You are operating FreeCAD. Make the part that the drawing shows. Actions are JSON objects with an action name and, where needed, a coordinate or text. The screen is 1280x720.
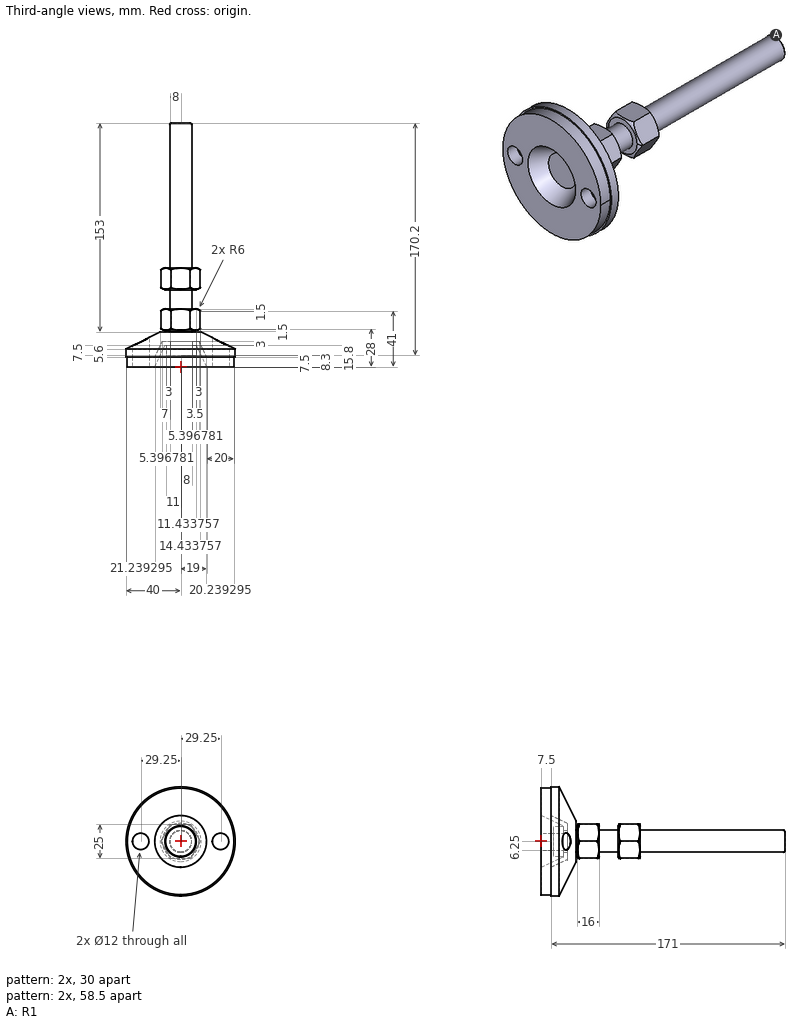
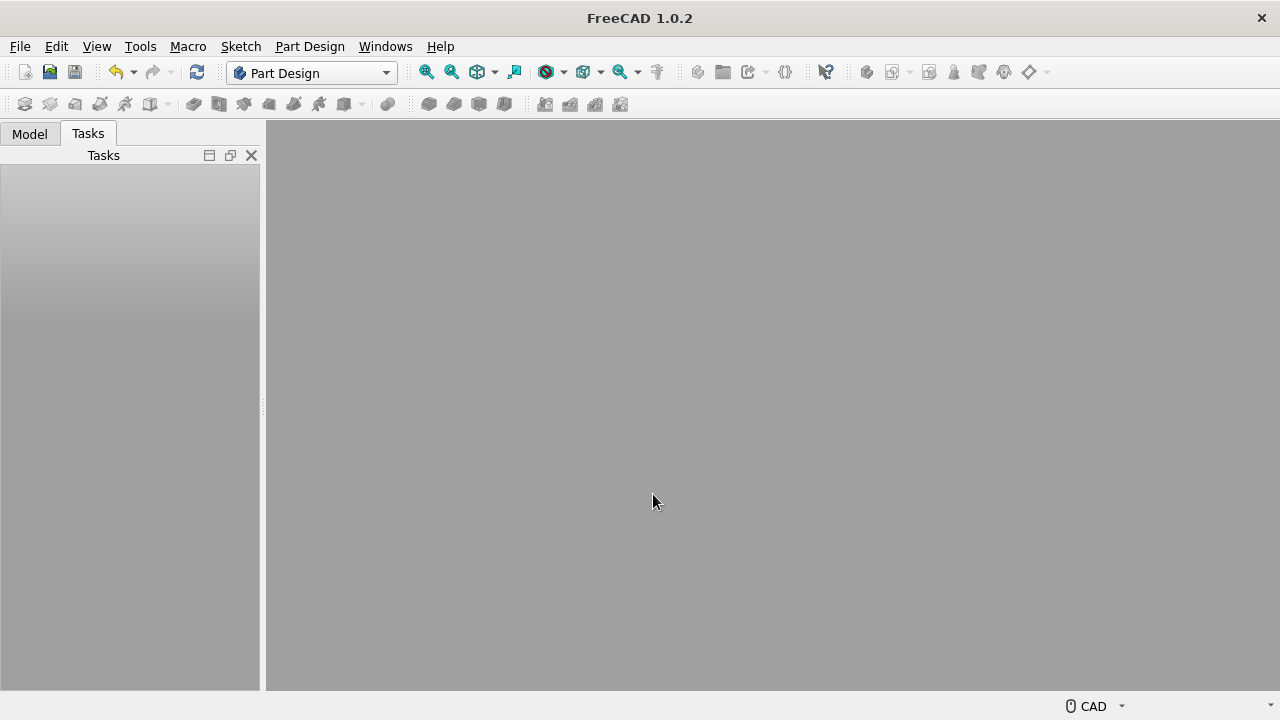
{"action": "left_click", "coordinate": [25, 72]}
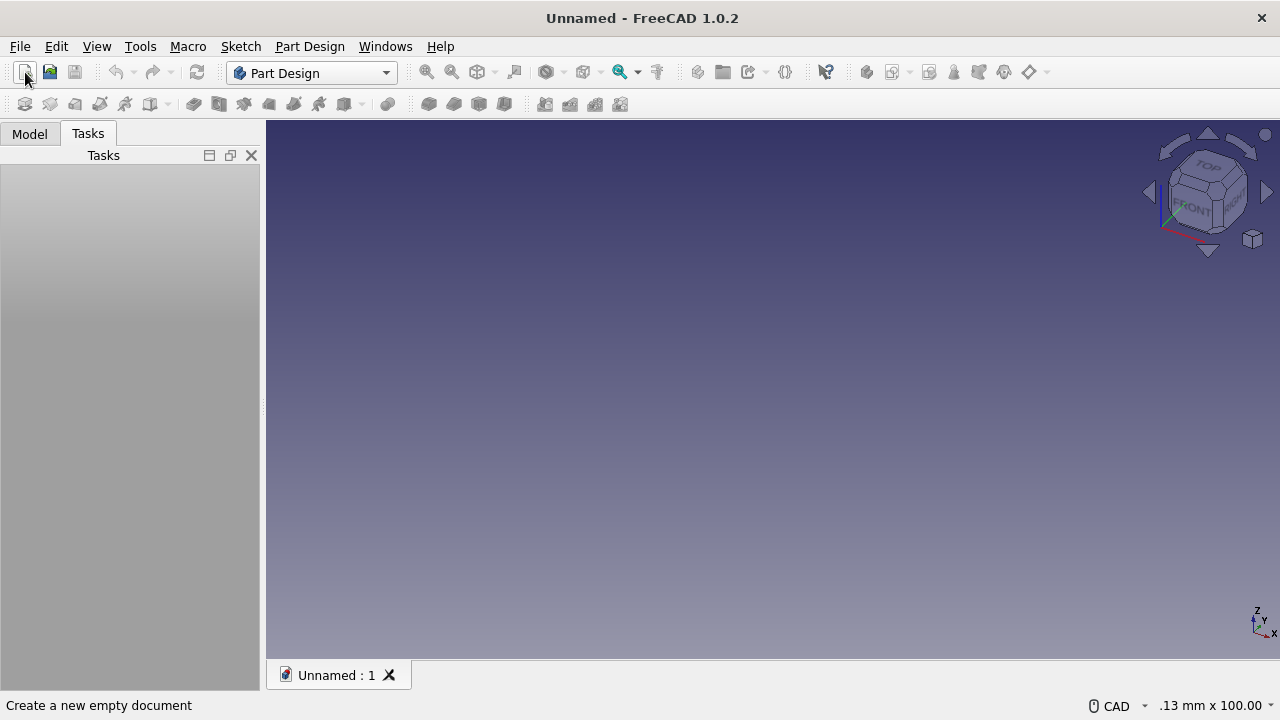
{"action": "left_click", "coordinate": [892, 72]}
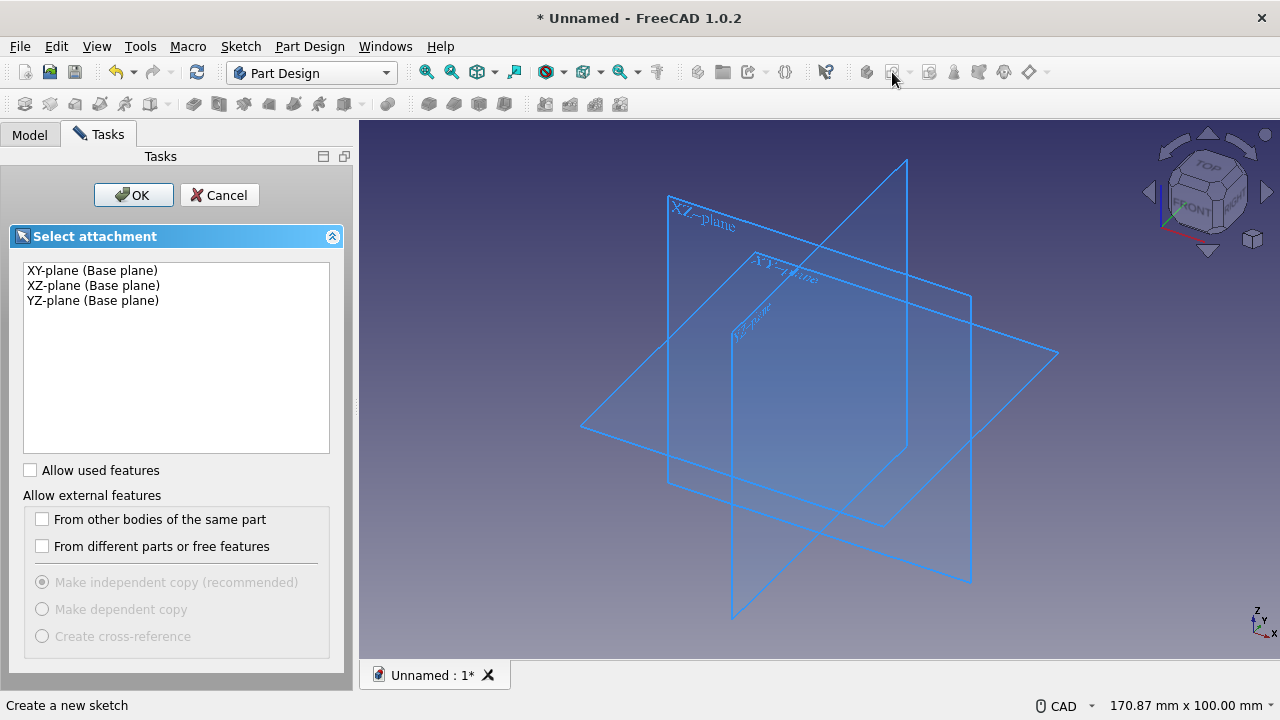
{"action": "left_click", "coordinate": [84, 270]}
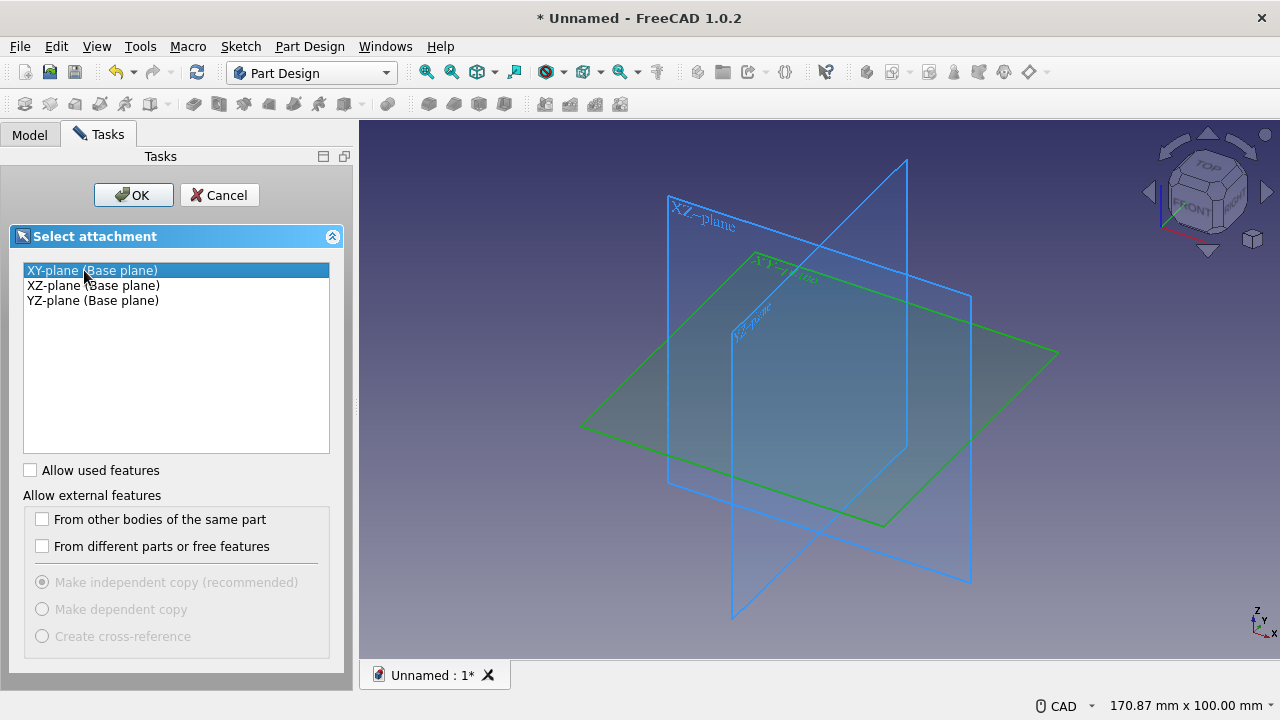
{"action": "left_click", "coordinate": [134, 195]}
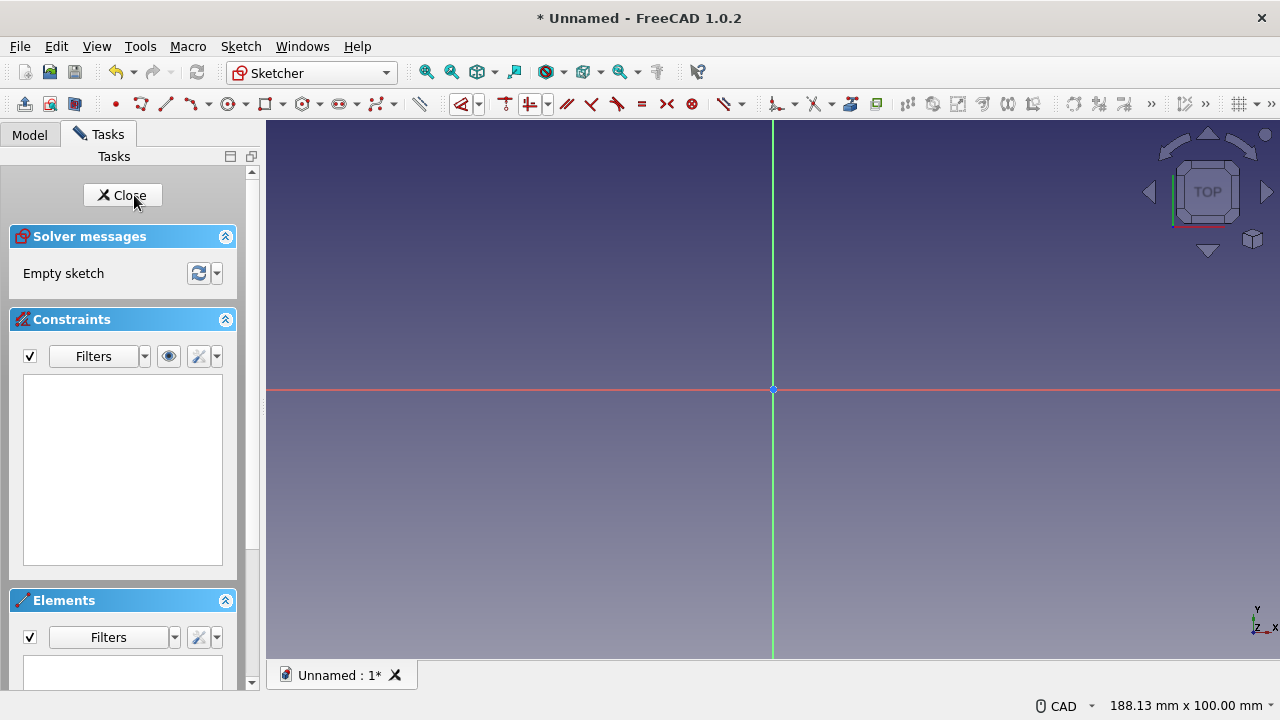
{"action": "scroll", "coordinate": [979, 309], "scroll_direction": "up", "scroll_amount": 5}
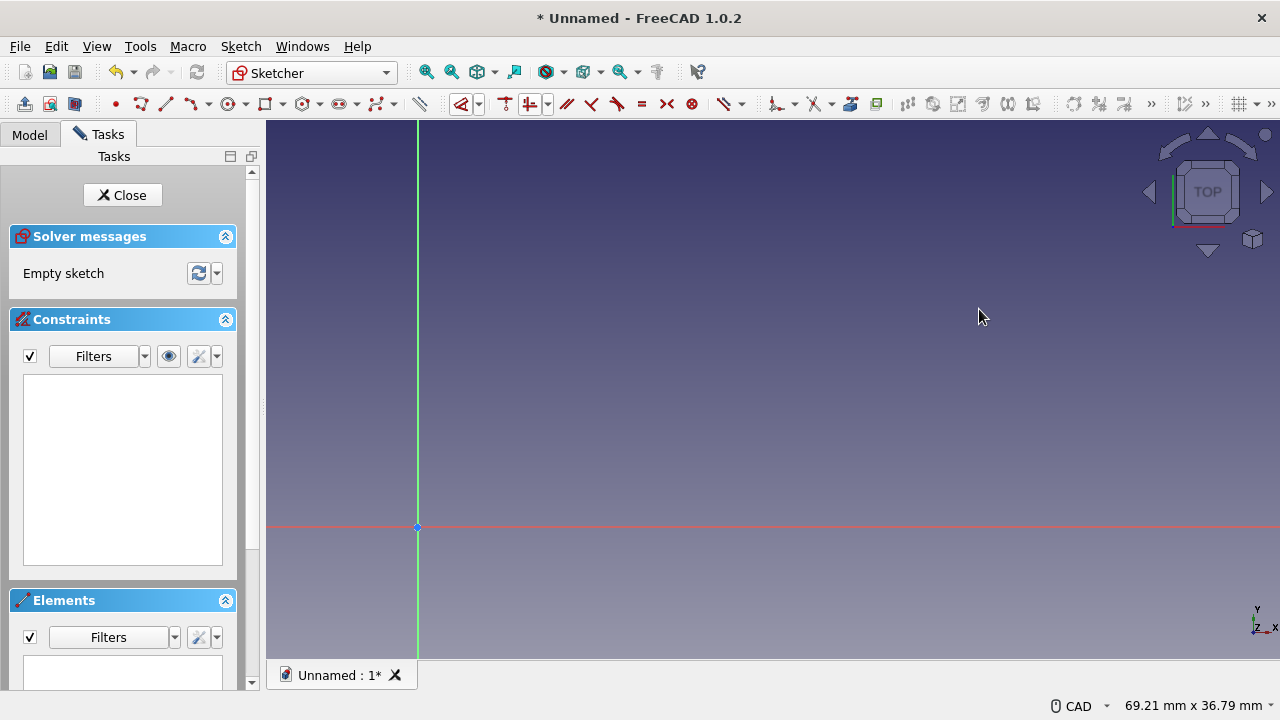
{"action": "left_click", "coordinate": [141, 104]}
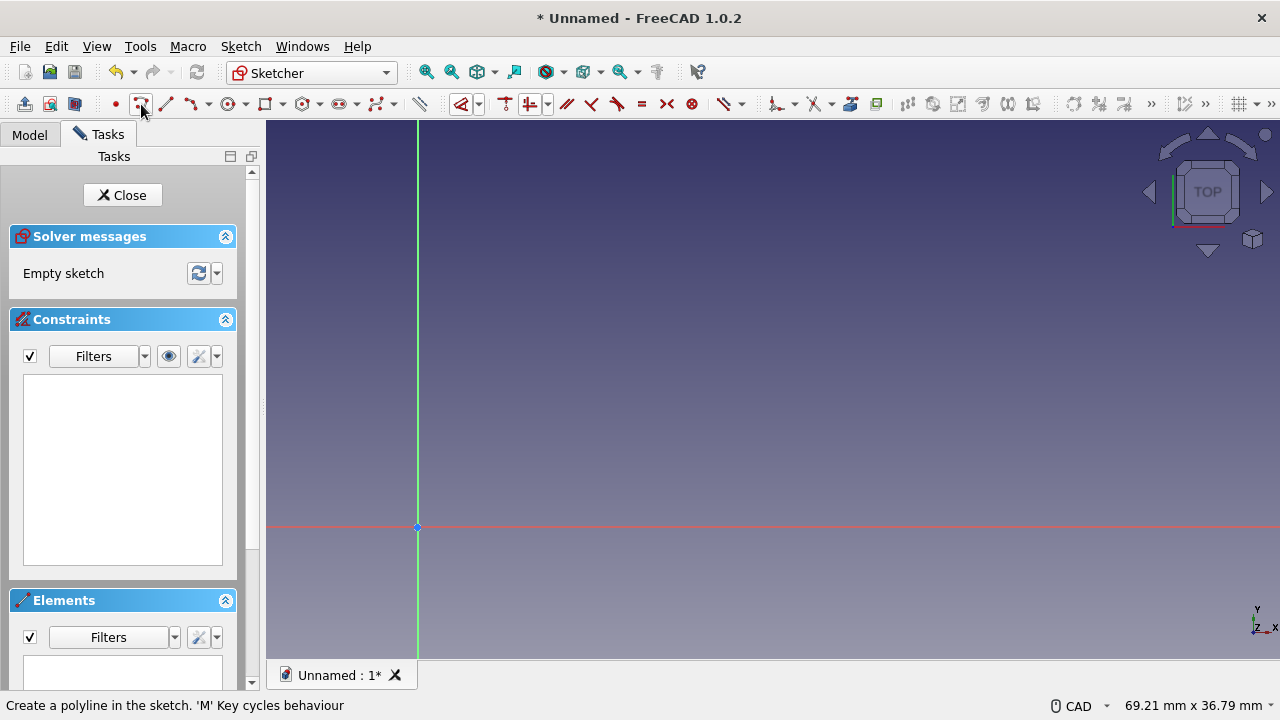
{"action": "left_click", "coordinate": [535, 296]}
{"action": "left_click", "coordinate": [586, 296]}
{"action": "left_click", "coordinate": [696, 527]}
{"action": "left_click", "coordinate": [989, 518]}
{"action": "left_click", "coordinate": [989, 417]}
{"action": "left_click", "coordinate": [693, 417]}
{"action": "left_click", "coordinate": [614, 252]}
{"action": "left_click", "coordinate": [535, 252]}
{"action": "left_click", "coordinate": [535, 297]}
{"action": "key", "text": "Escape"}
{"action": "key", "text": "Escape"}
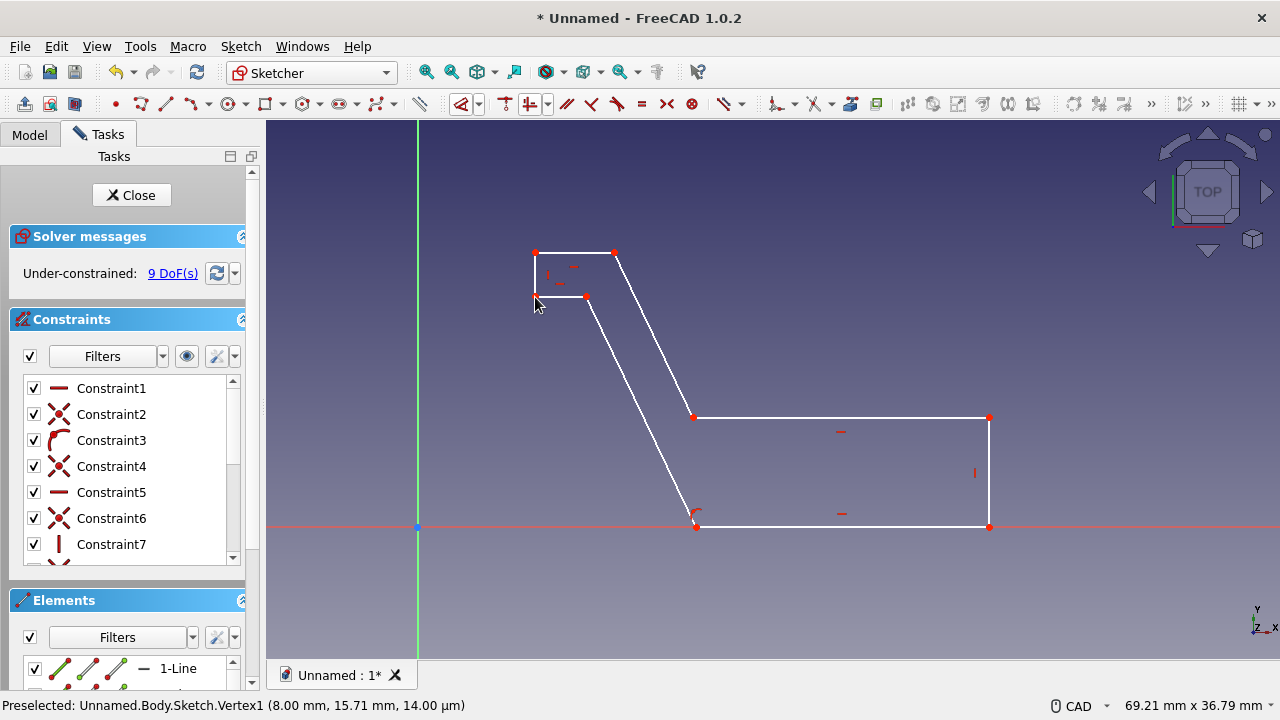
{"action": "left_click", "coordinate": [460, 104]}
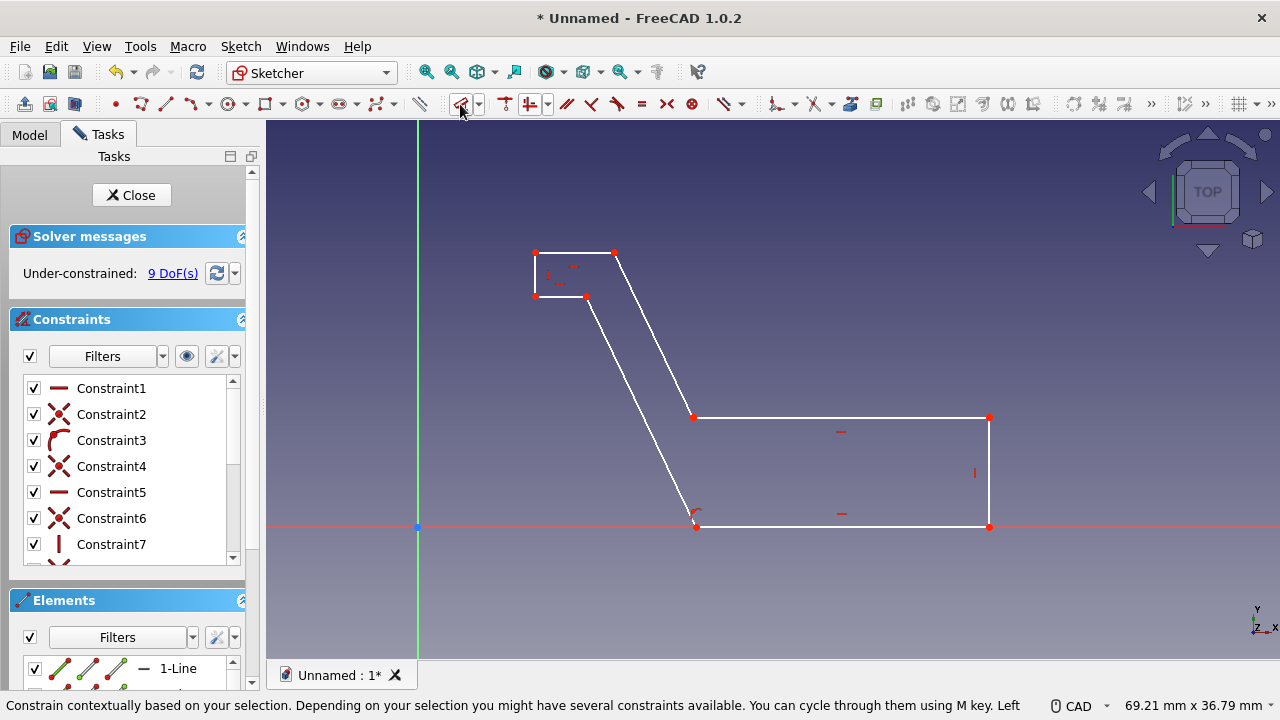
{"action": "left_click", "coordinate": [535, 266]}
{"action": "left_click", "coordinate": [501, 275]}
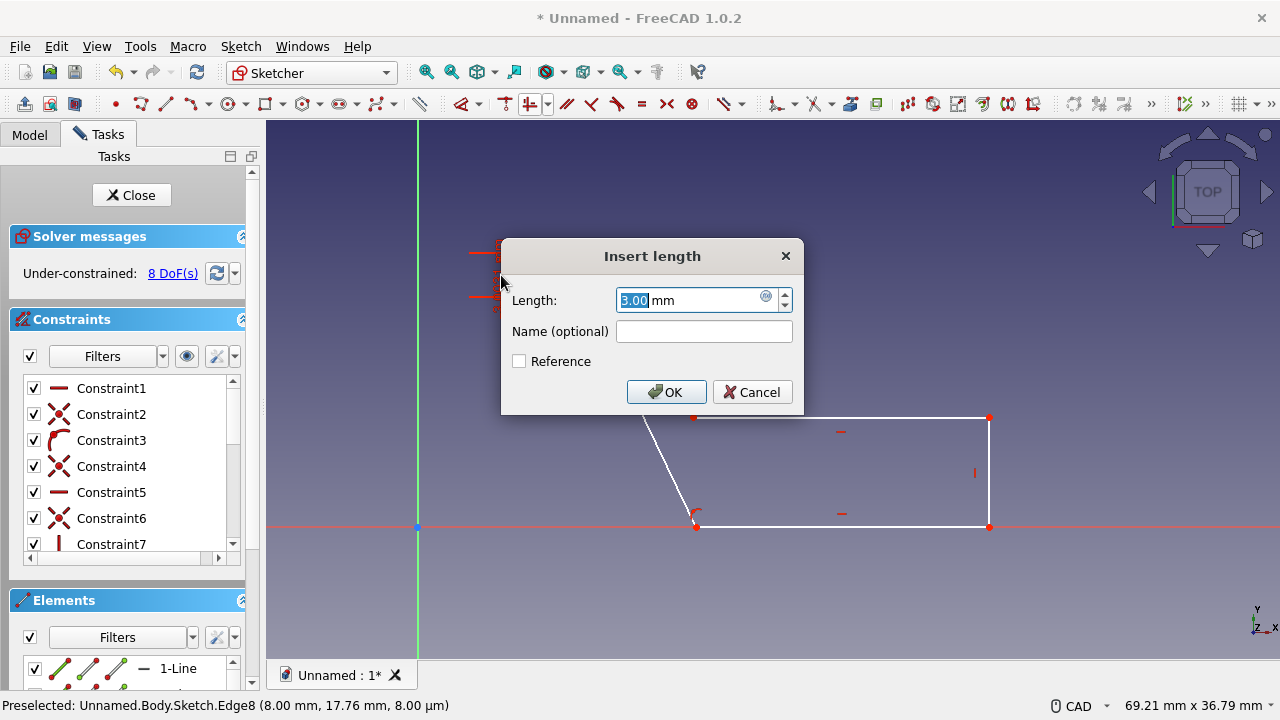
{"action": "type", "text": "3"}
{"action": "key", "text": "Return"}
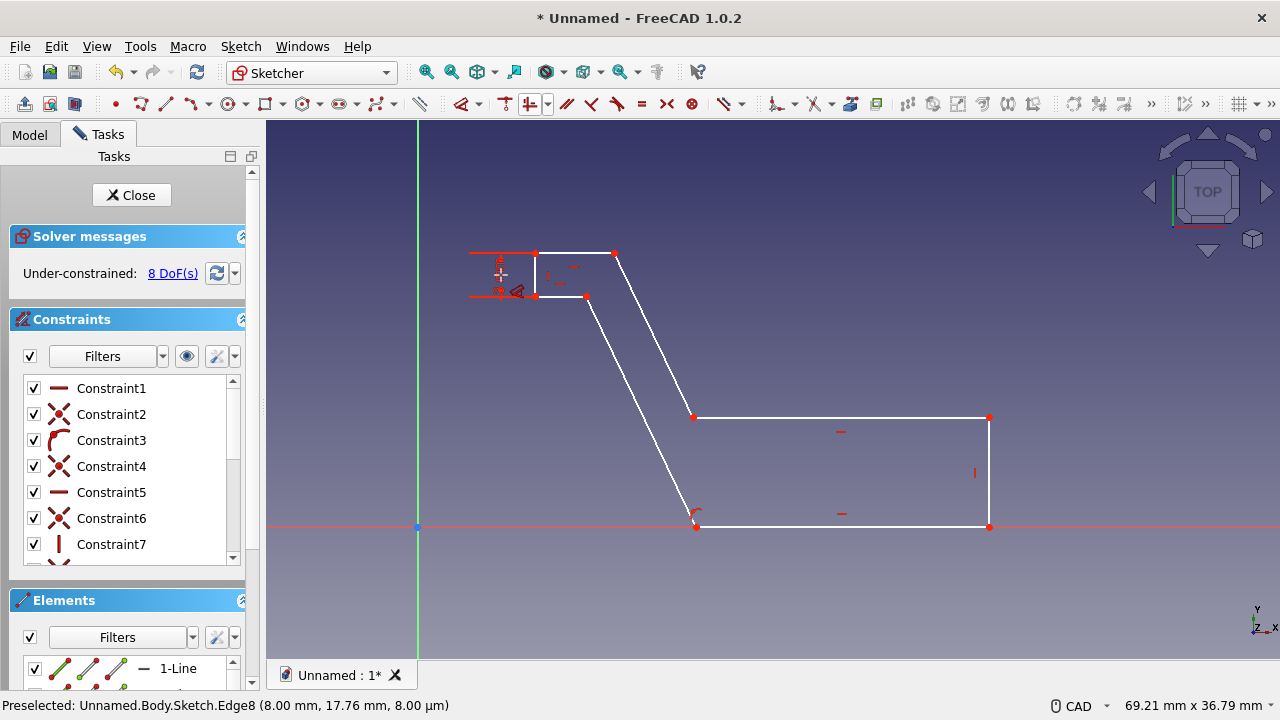
{"action": "left_click", "coordinate": [784, 527]}
{"action": "left_click", "coordinate": [843, 561]}